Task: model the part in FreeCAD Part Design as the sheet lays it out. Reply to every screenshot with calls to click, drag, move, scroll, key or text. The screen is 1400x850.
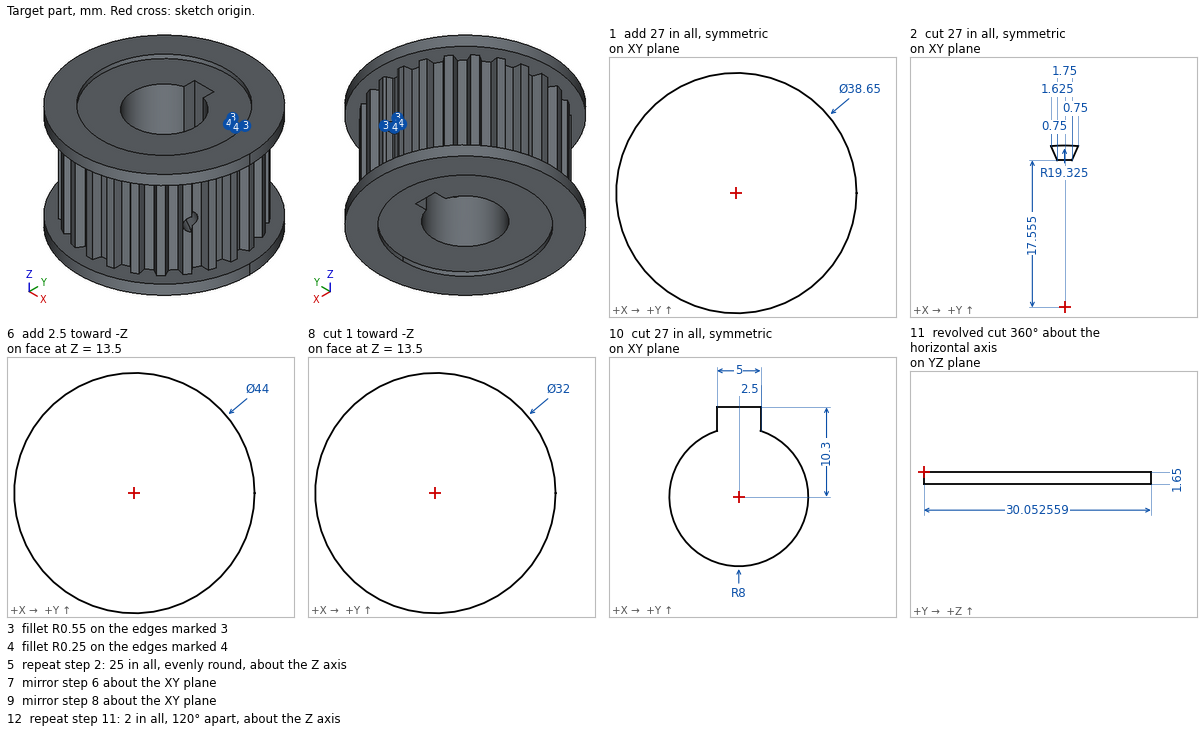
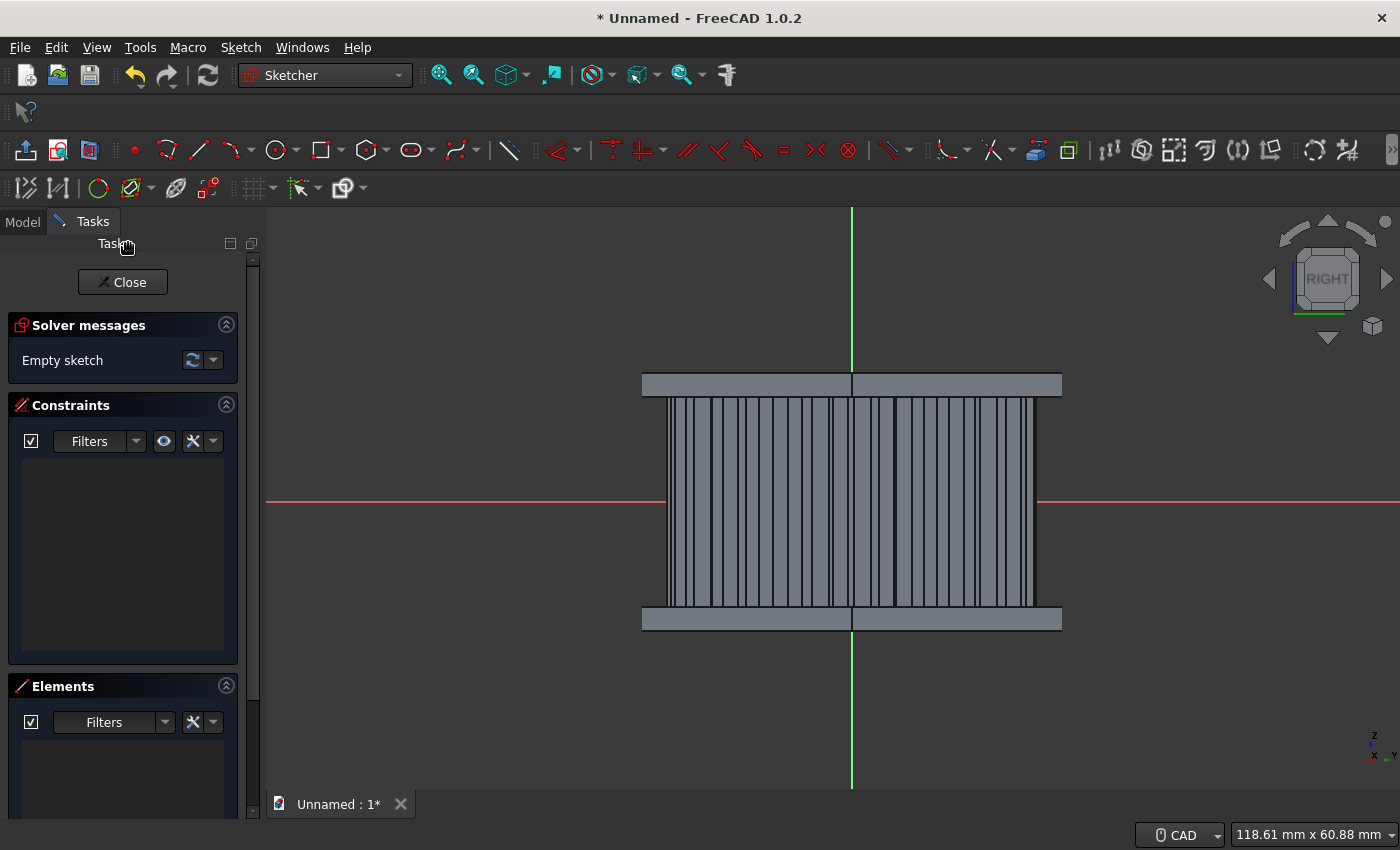
click(90, 150)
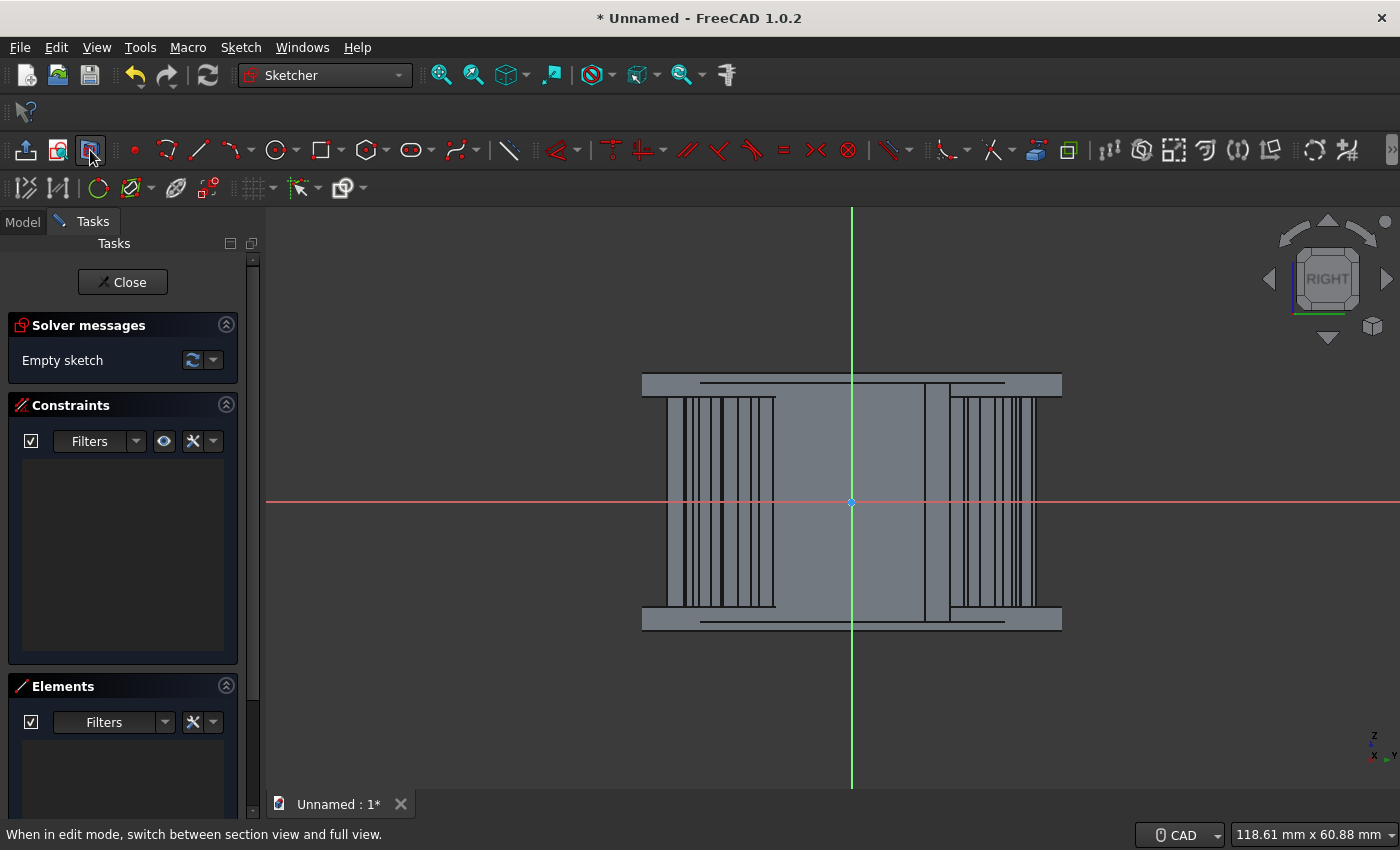
scroll(1184, 520, up, 4)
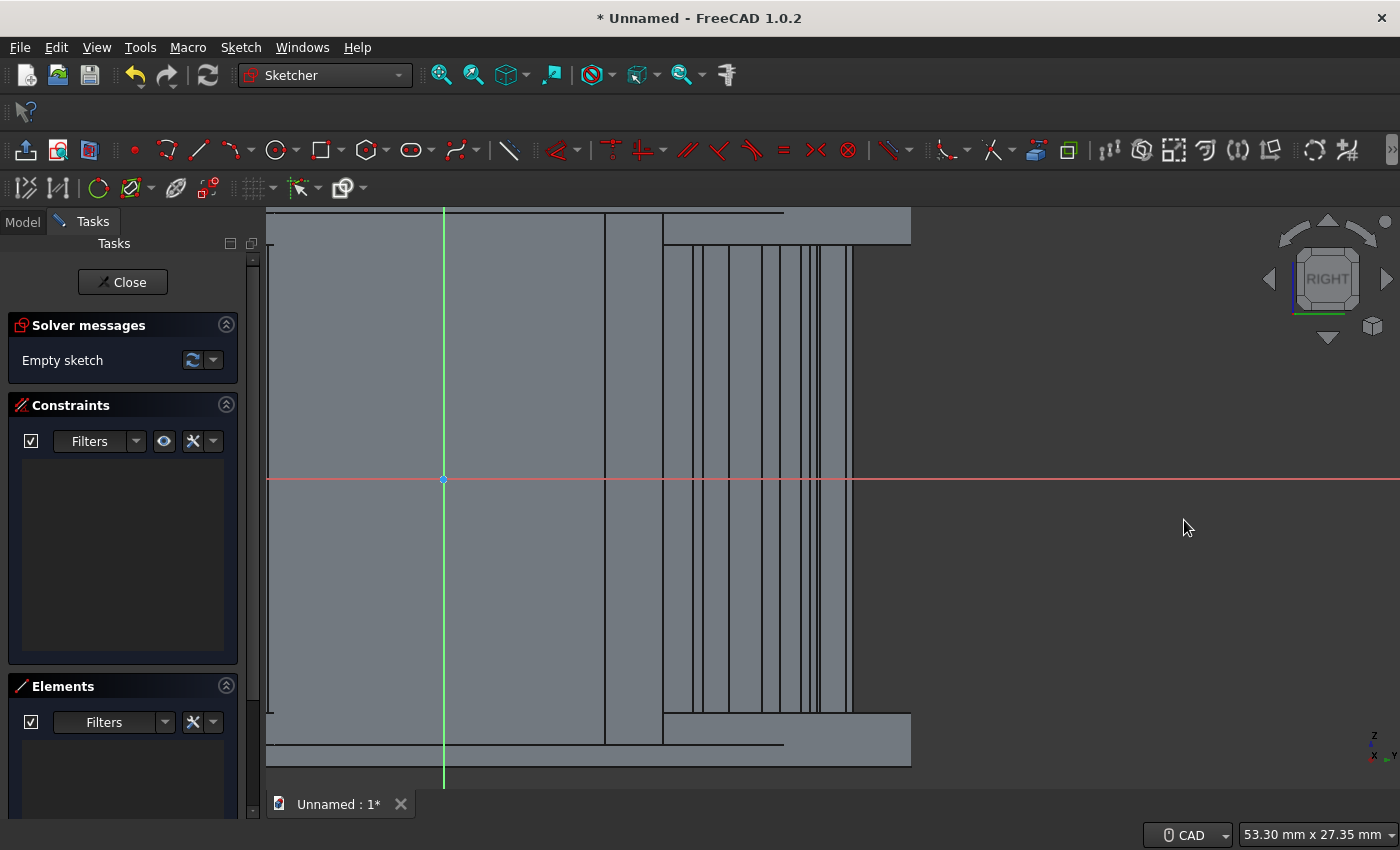
click(322, 150)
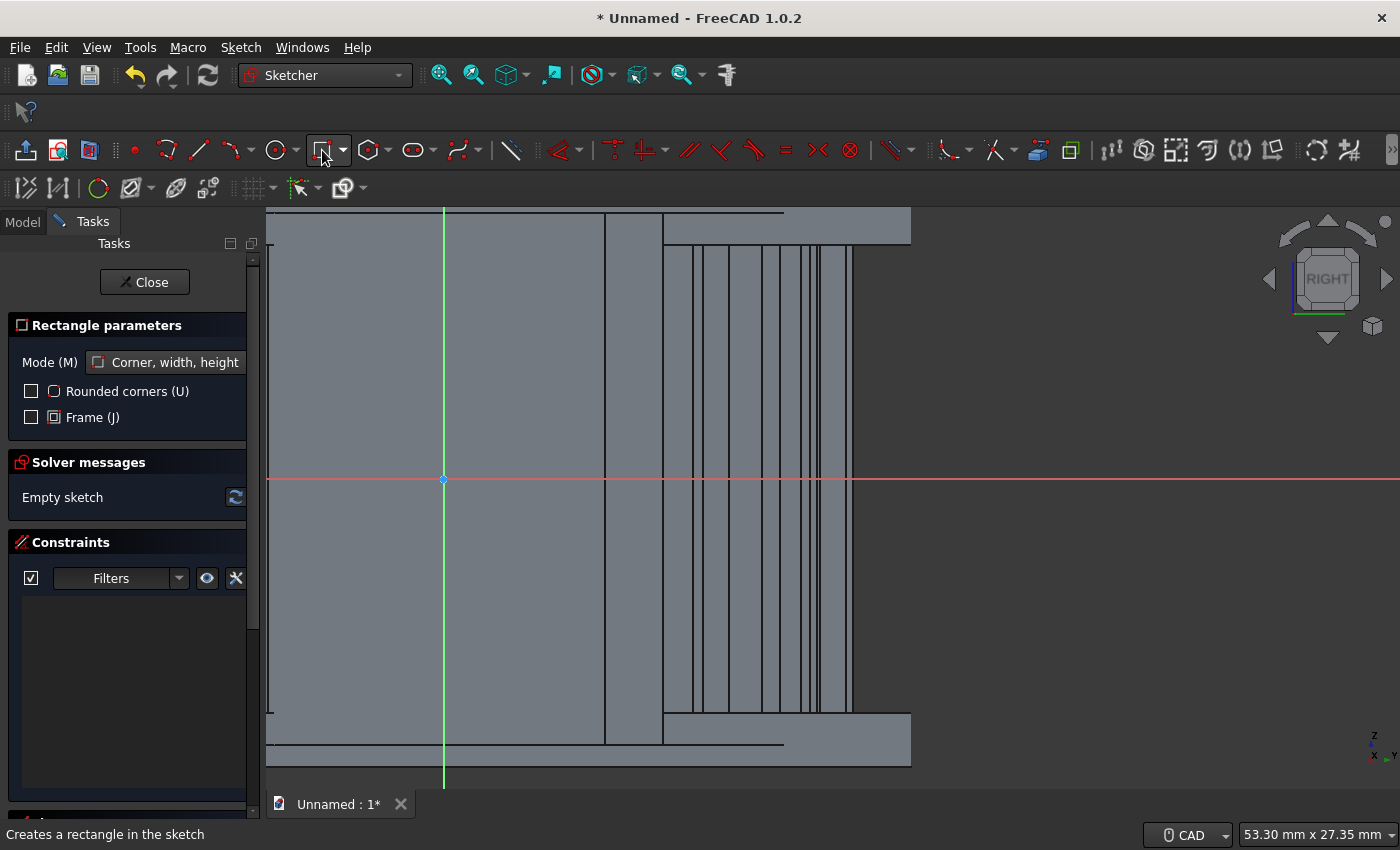
click(444, 479)
move(1083, 514)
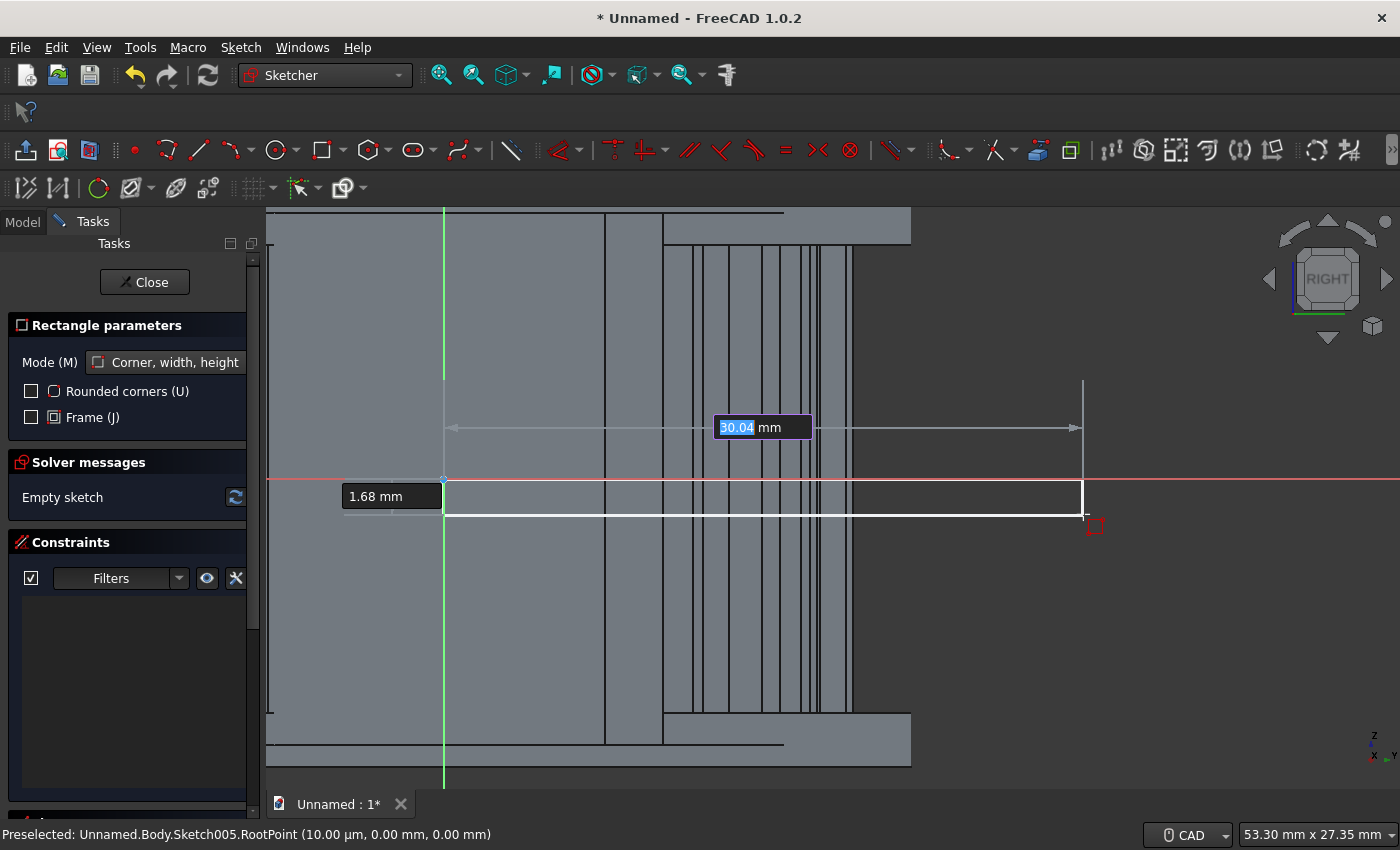
text(30.052559)
key(Tab)
text(1.65)
key(Return)
key(Escape)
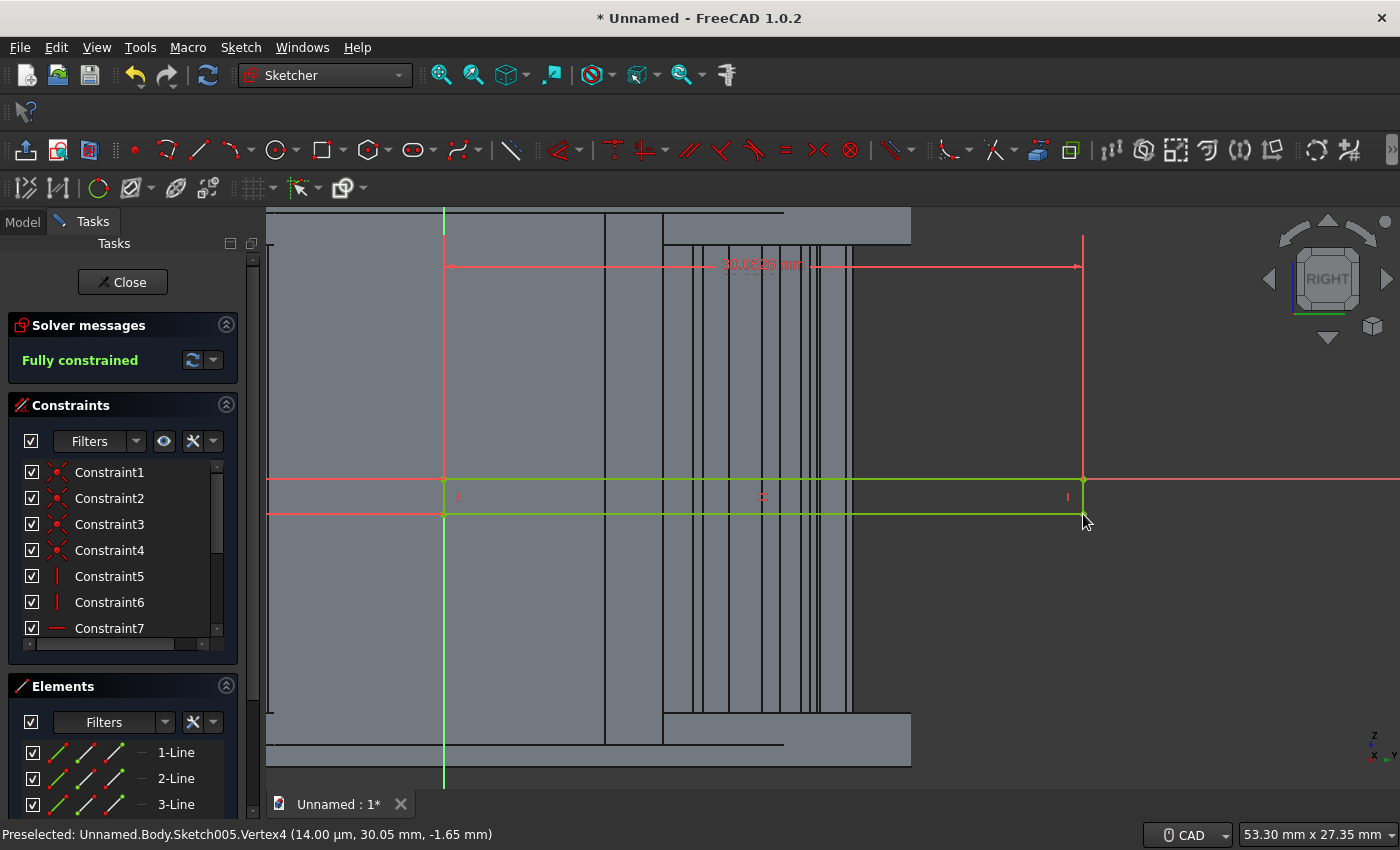
click(123, 282)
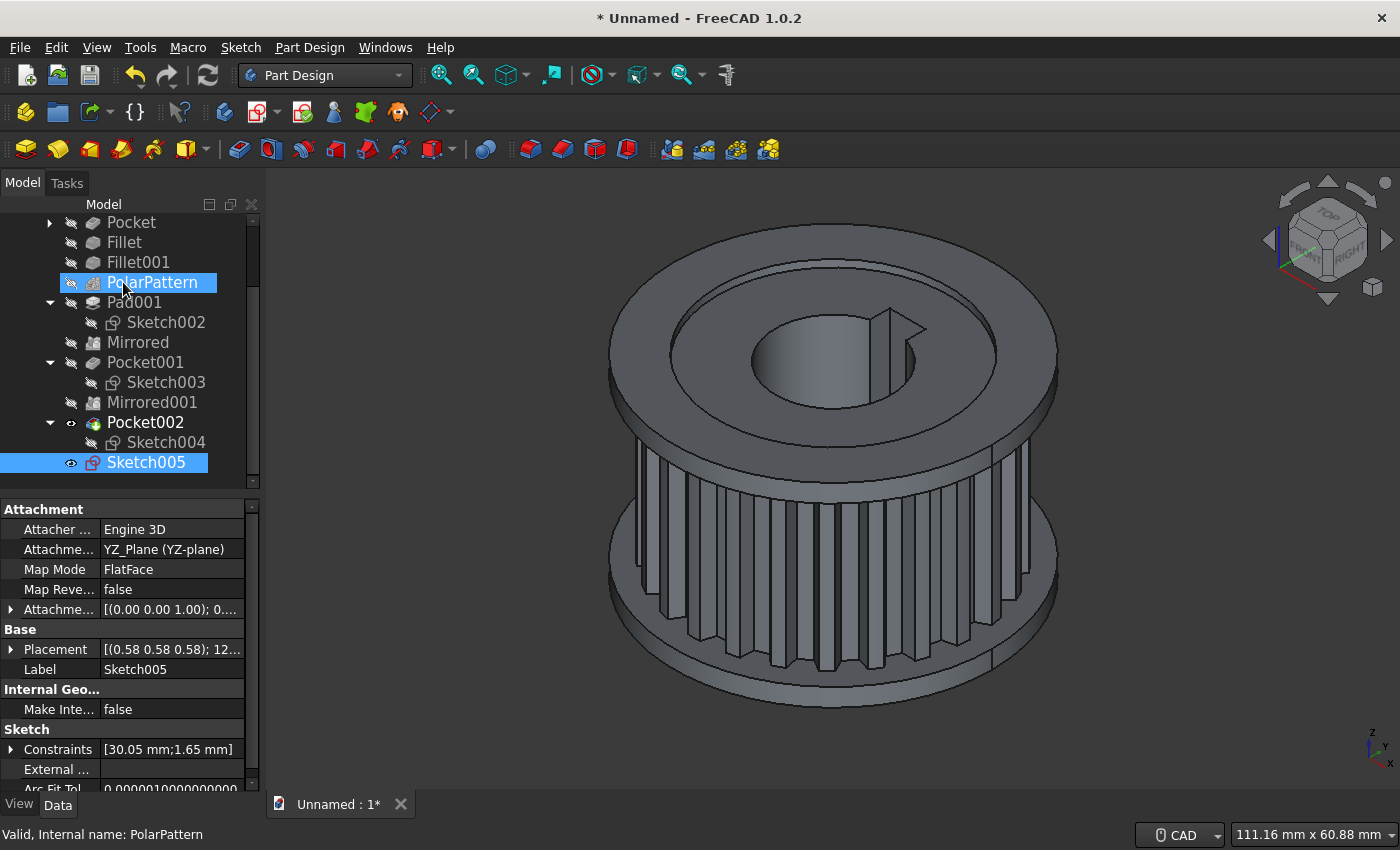
click(304, 150)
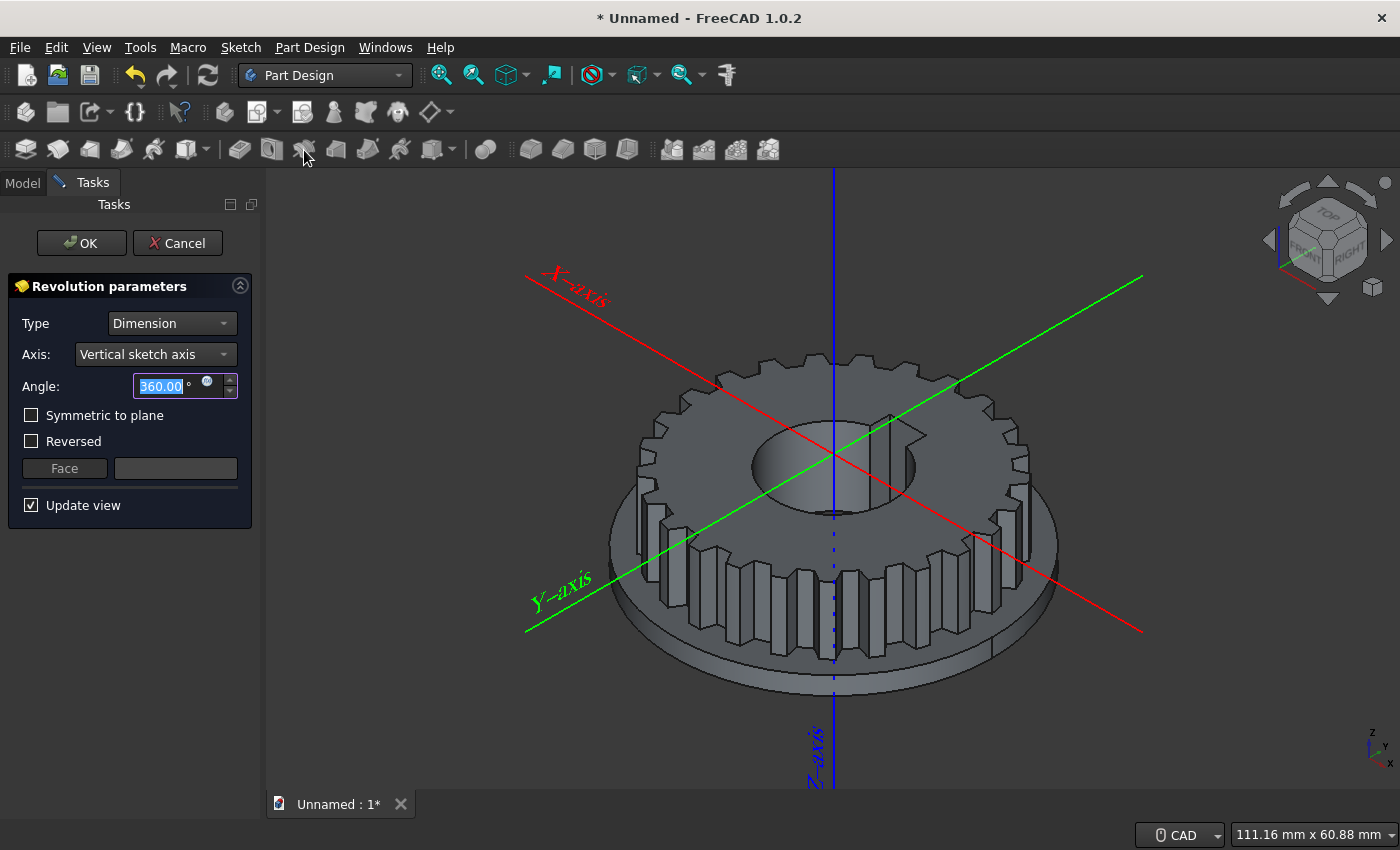
click(156, 354)